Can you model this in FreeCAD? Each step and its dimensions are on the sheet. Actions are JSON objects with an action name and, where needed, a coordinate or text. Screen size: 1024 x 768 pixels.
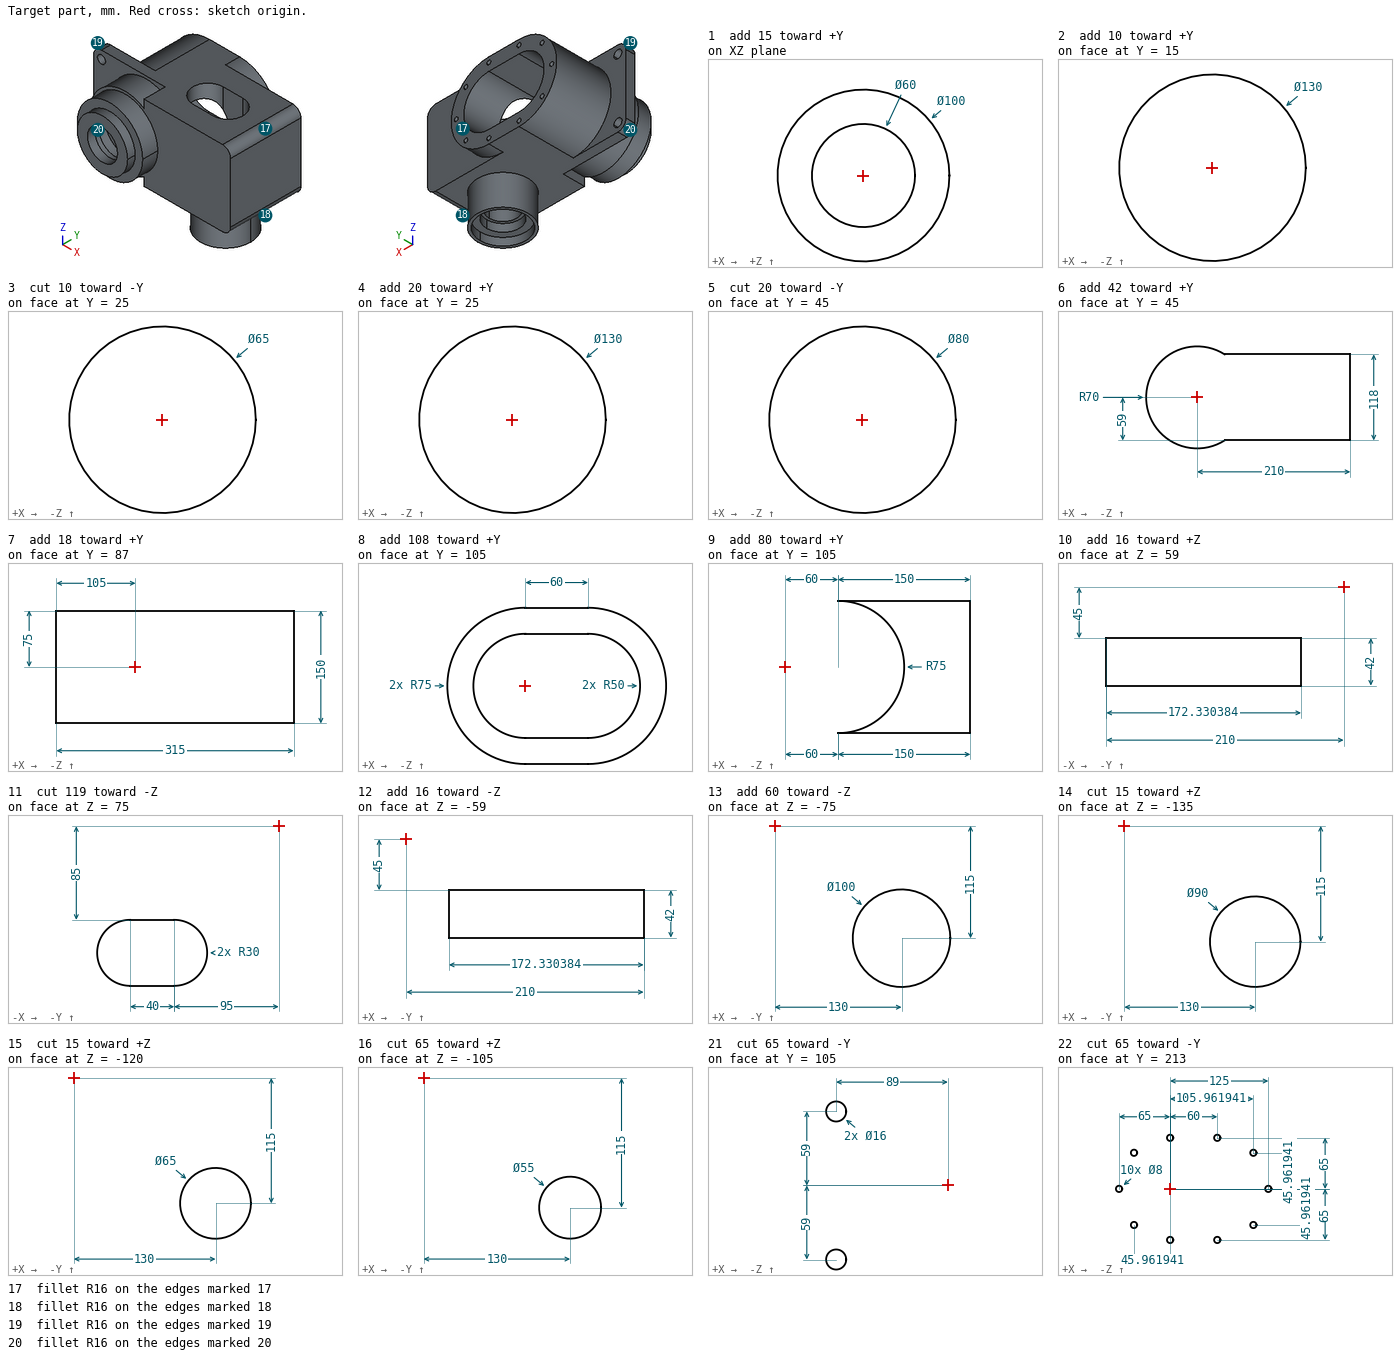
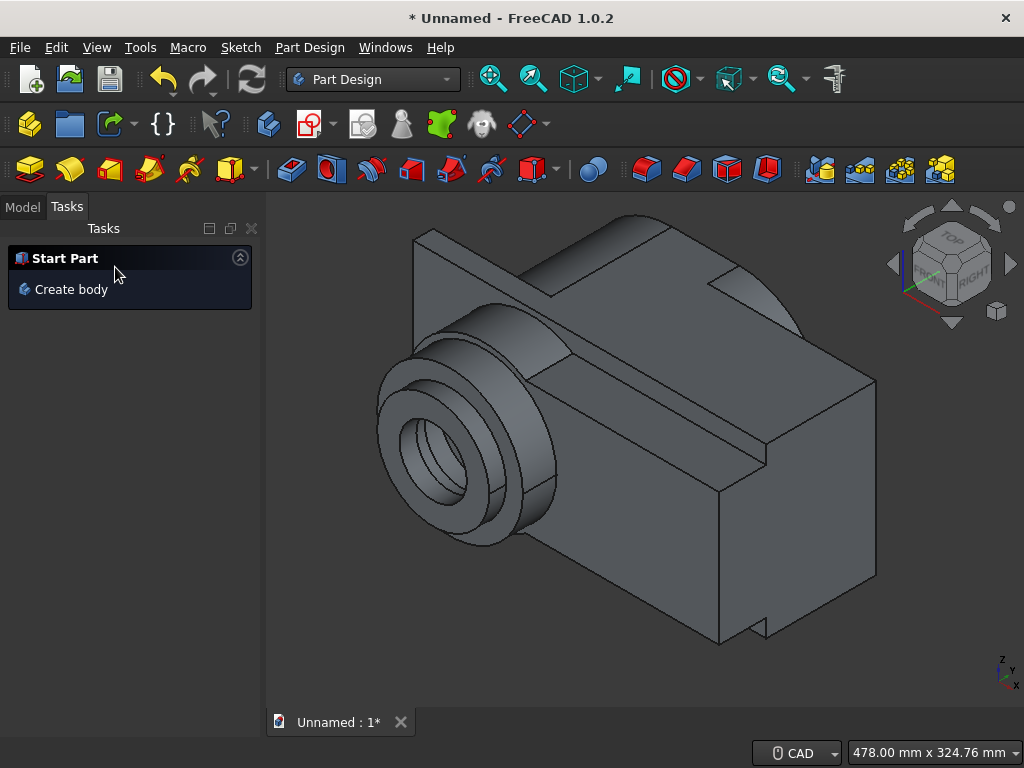
{"action": "left_click", "coordinate": [494, 80]}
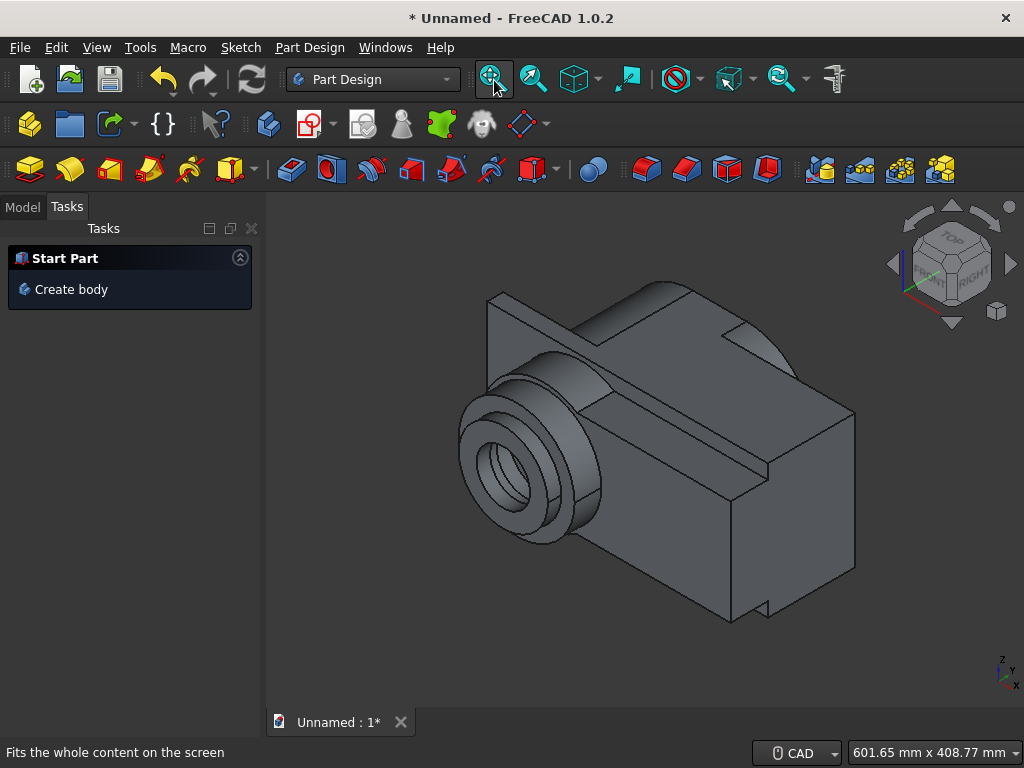
{"action": "left_click", "coordinate": [716, 471]}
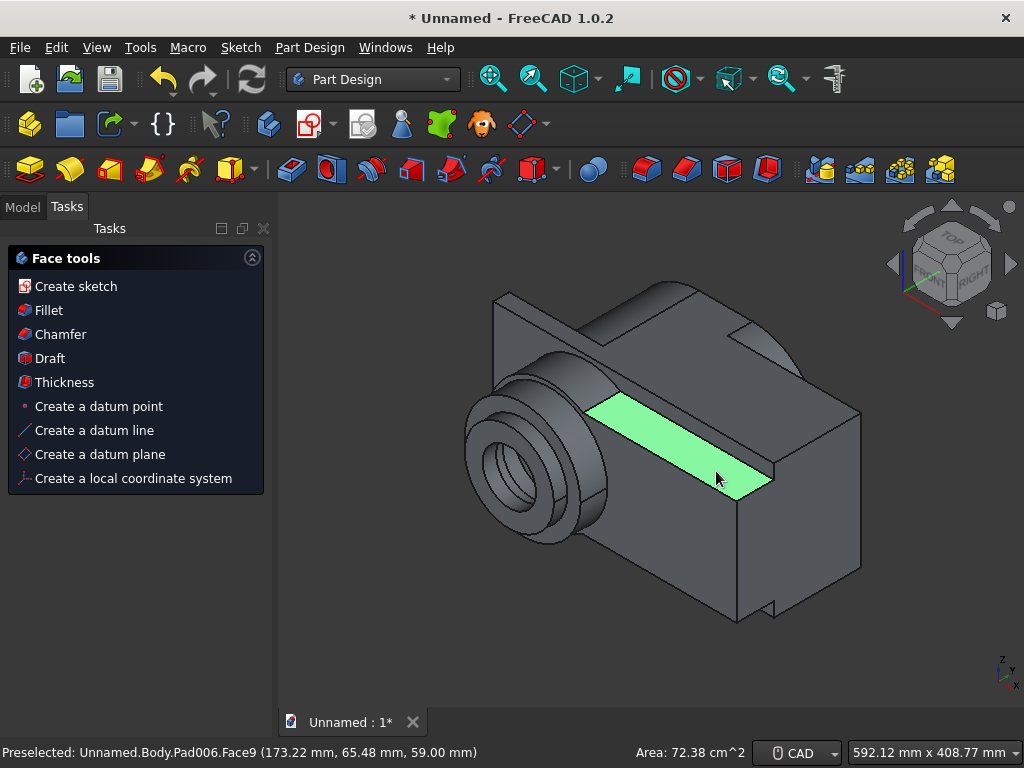
{"action": "left_click", "coordinate": [310, 124]}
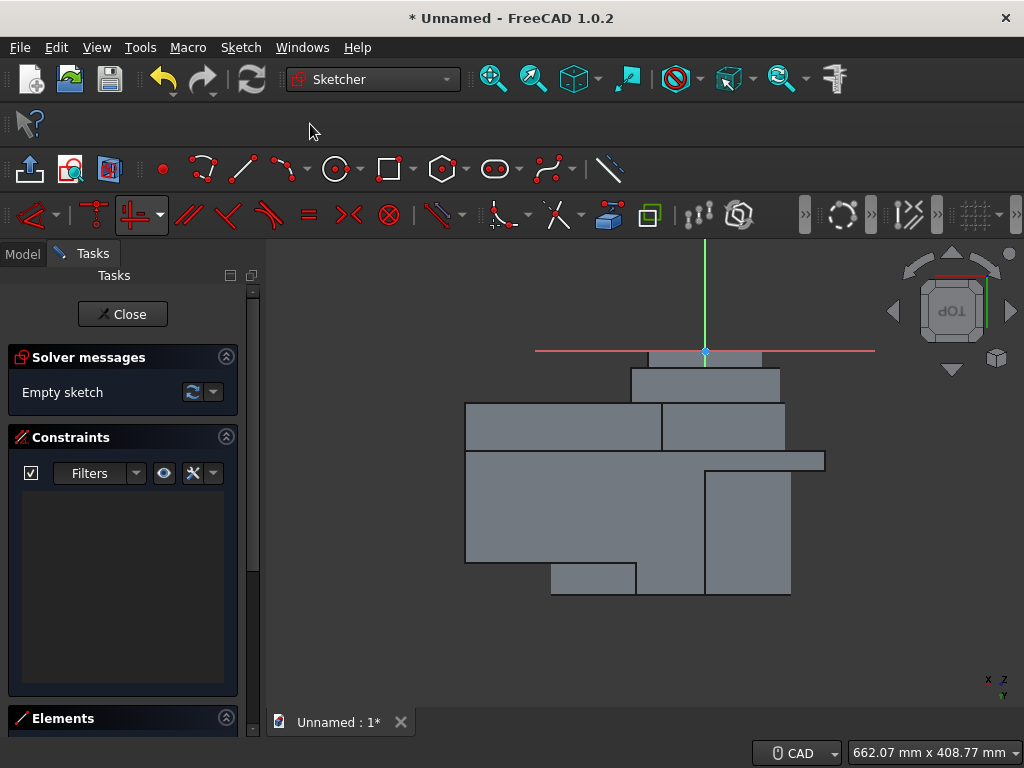
{"action": "left_click", "coordinate": [110, 170]}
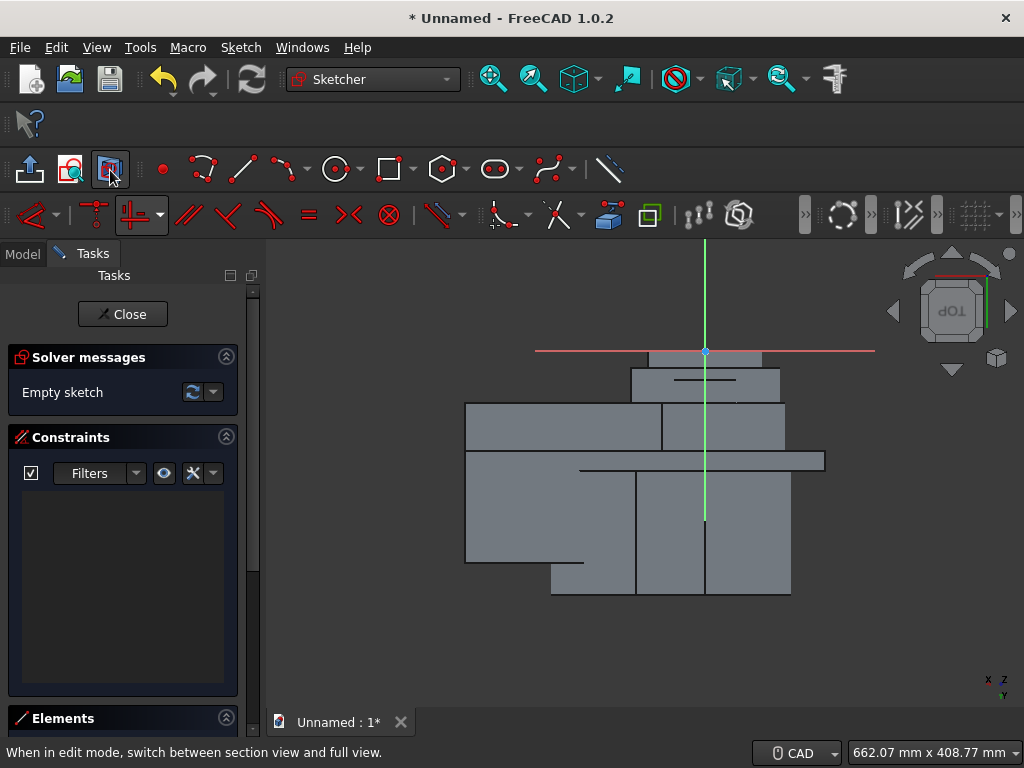
{"action": "scroll", "coordinate": [595, 313], "scroll_direction": "up", "scroll_amount": 3}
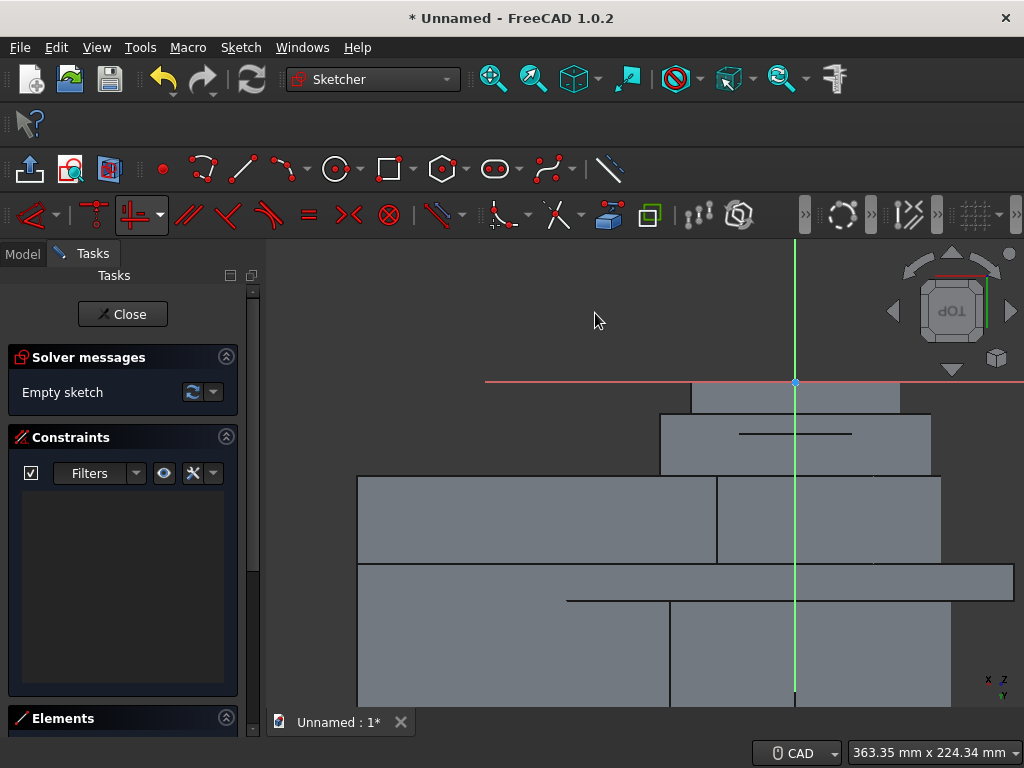
{"action": "left_click", "coordinate": [390, 170]}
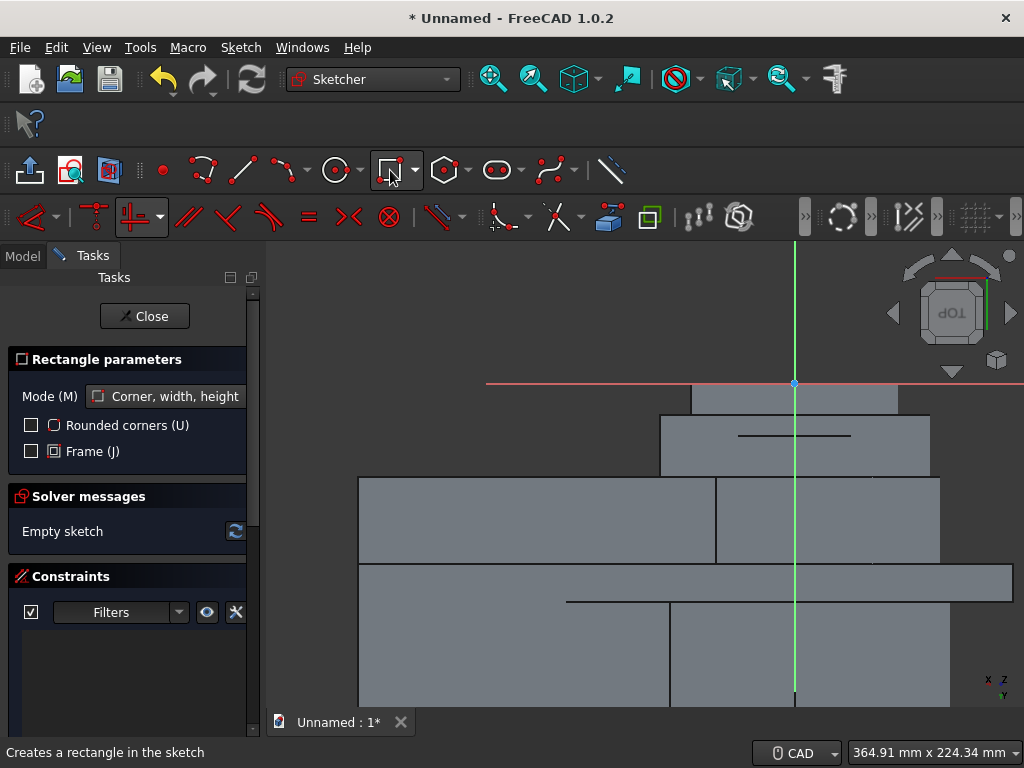
{"action": "left_click", "coordinate": [358, 477]}
{"action": "mouse_move", "coordinate": [716, 564]}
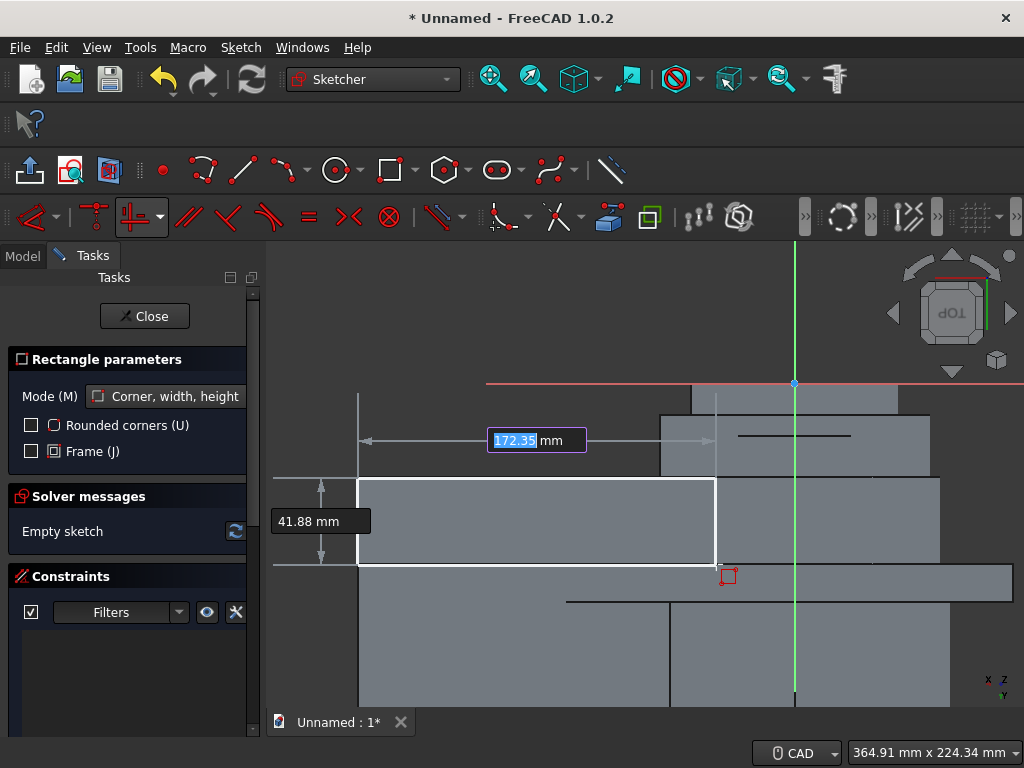
{"action": "type", "text": "172.330384"}
{"action": "key", "text": "Tab"}
{"action": "type", "text": "42"}
{"action": "key", "text": "Return"}
{"action": "key", "text": "Escape"}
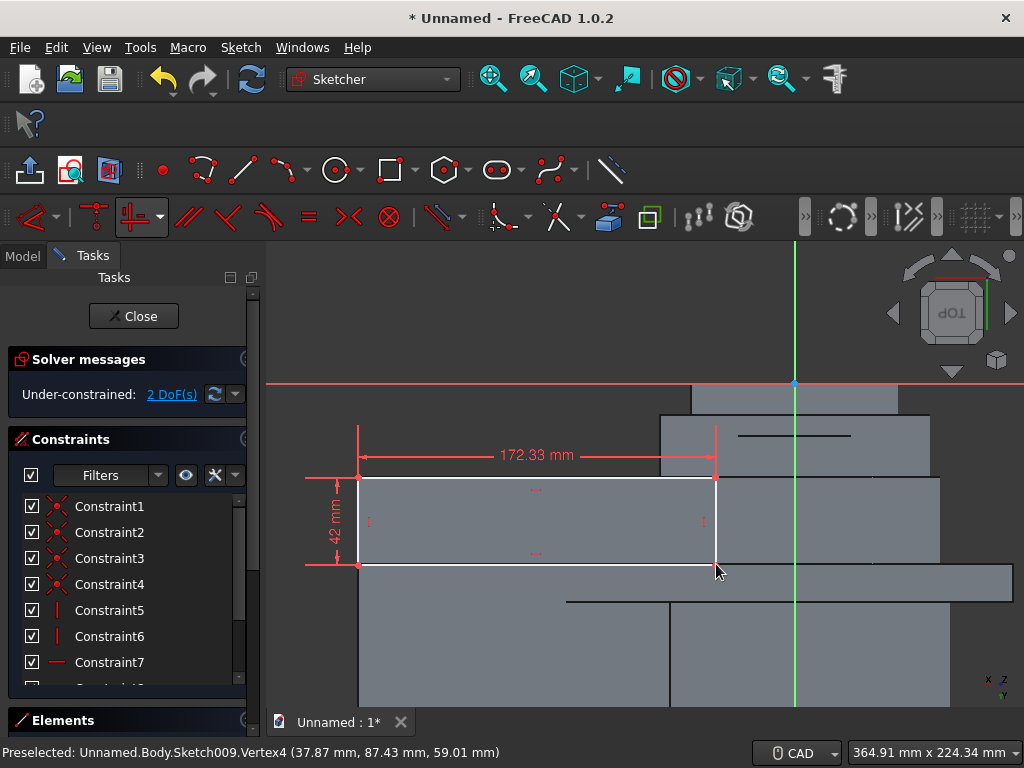
{"action": "left_click", "coordinate": [32, 218]}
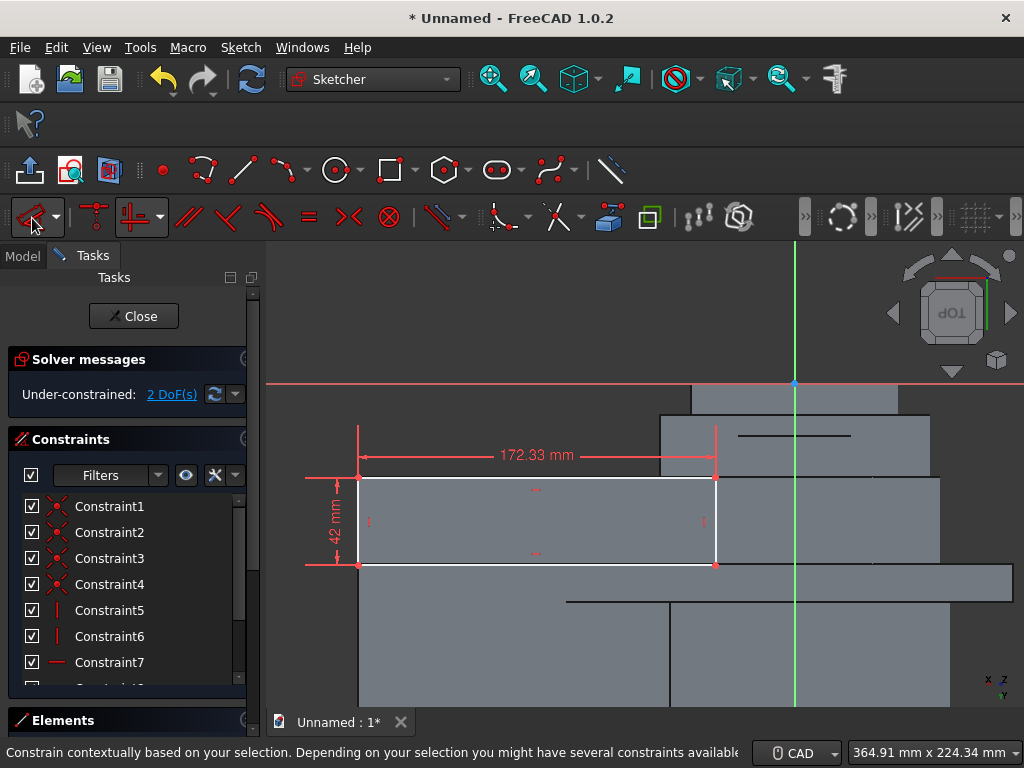
{"action": "left_click", "coordinate": [358, 478]}
{"action": "left_click", "coordinate": [324, 431]}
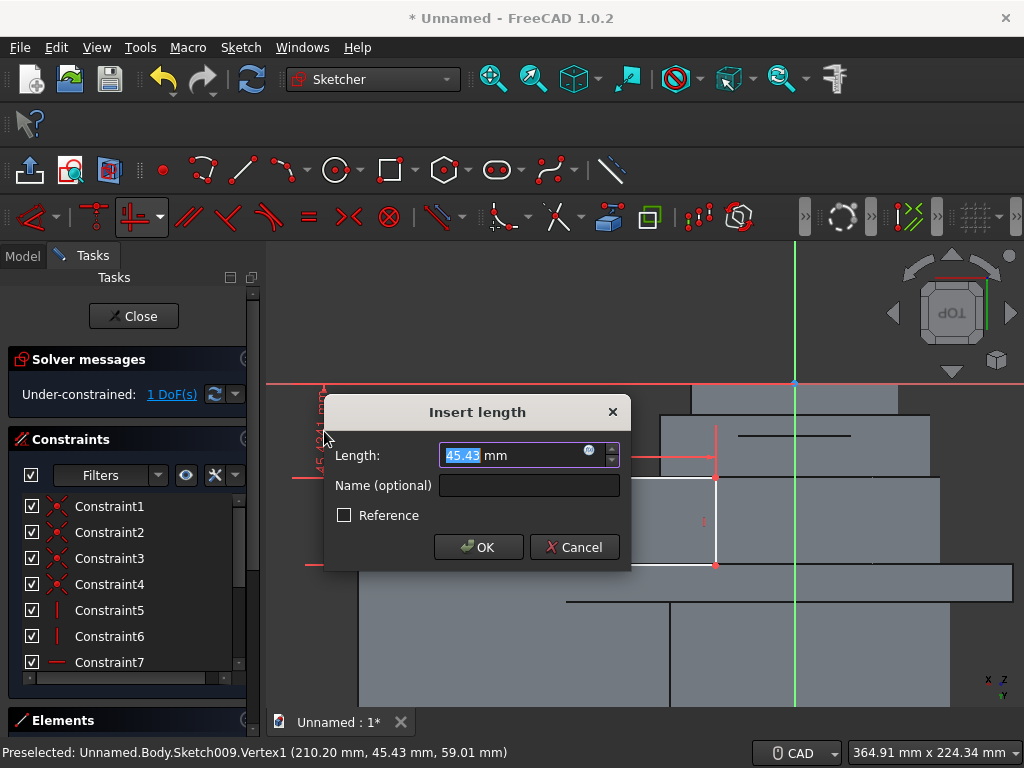
{"action": "type", "text": "45"}
{"action": "key", "text": "Return"}